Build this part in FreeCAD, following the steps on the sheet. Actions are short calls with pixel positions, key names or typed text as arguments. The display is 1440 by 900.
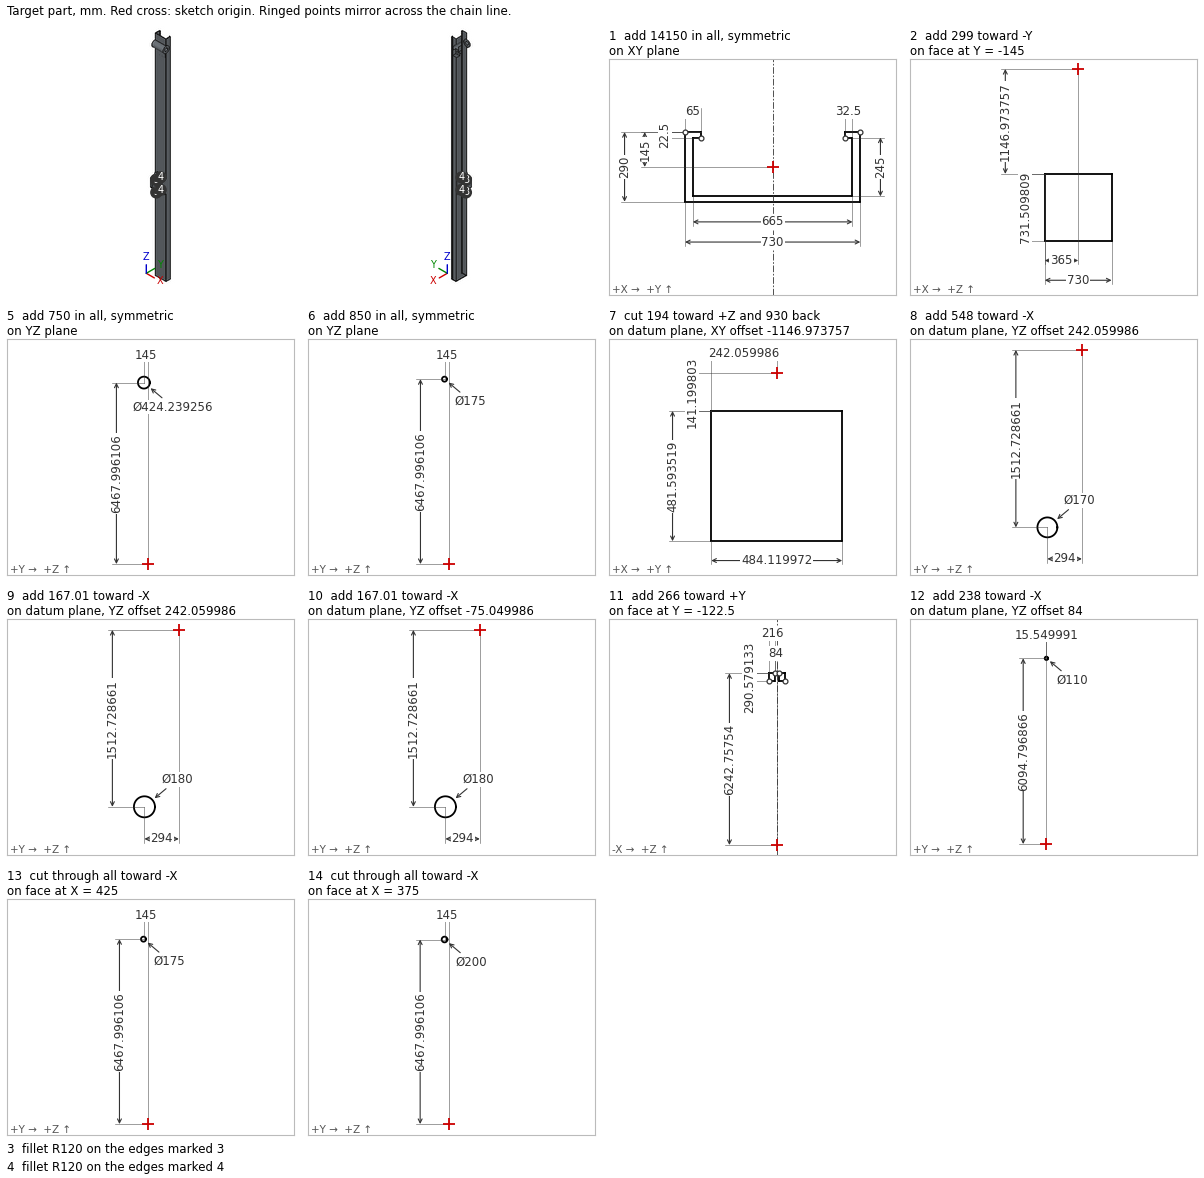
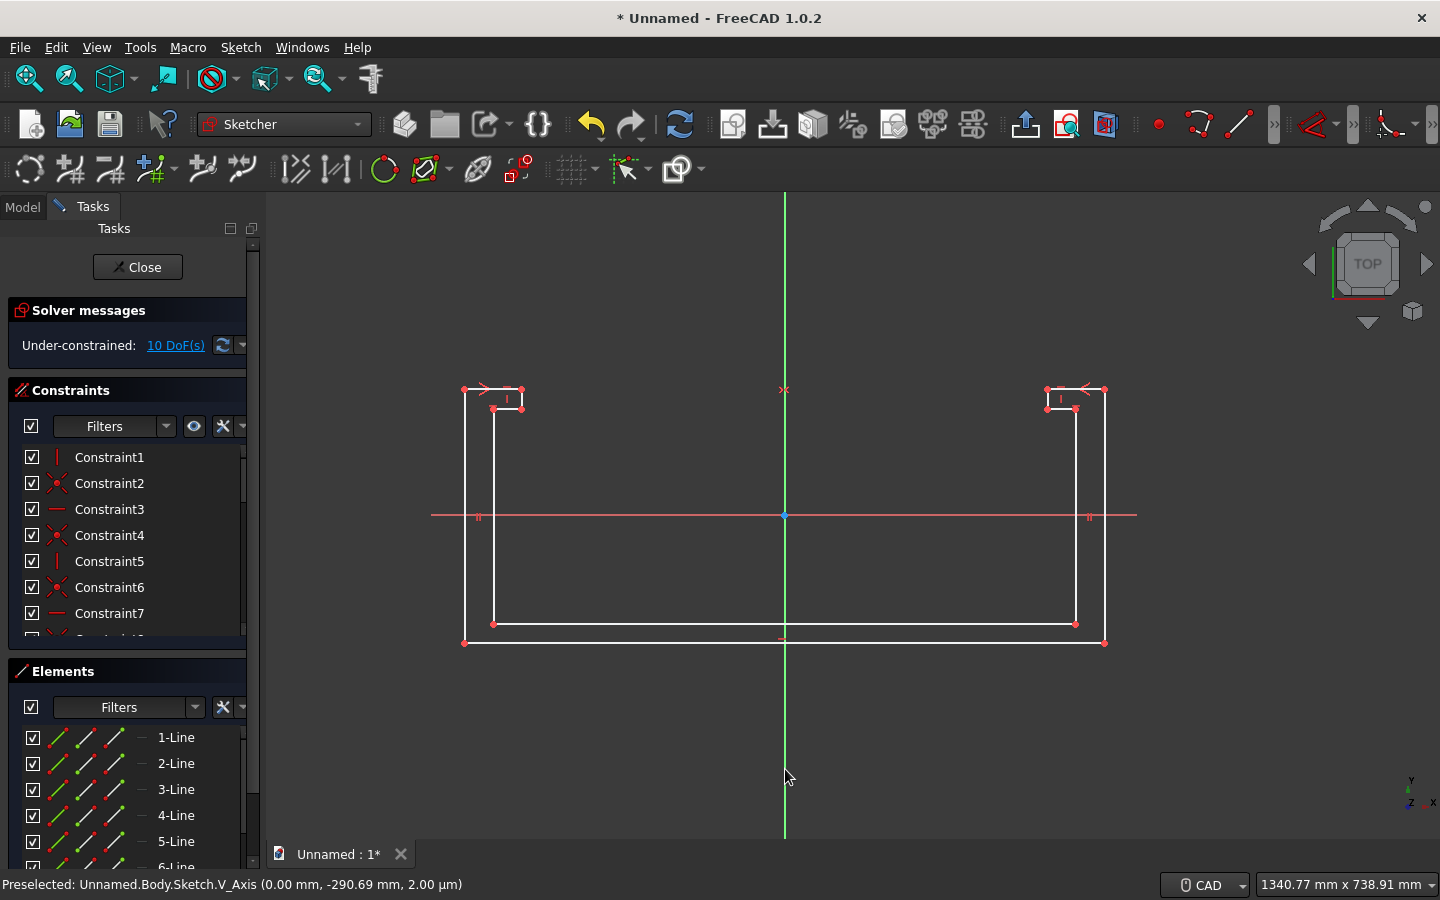
click(522, 409)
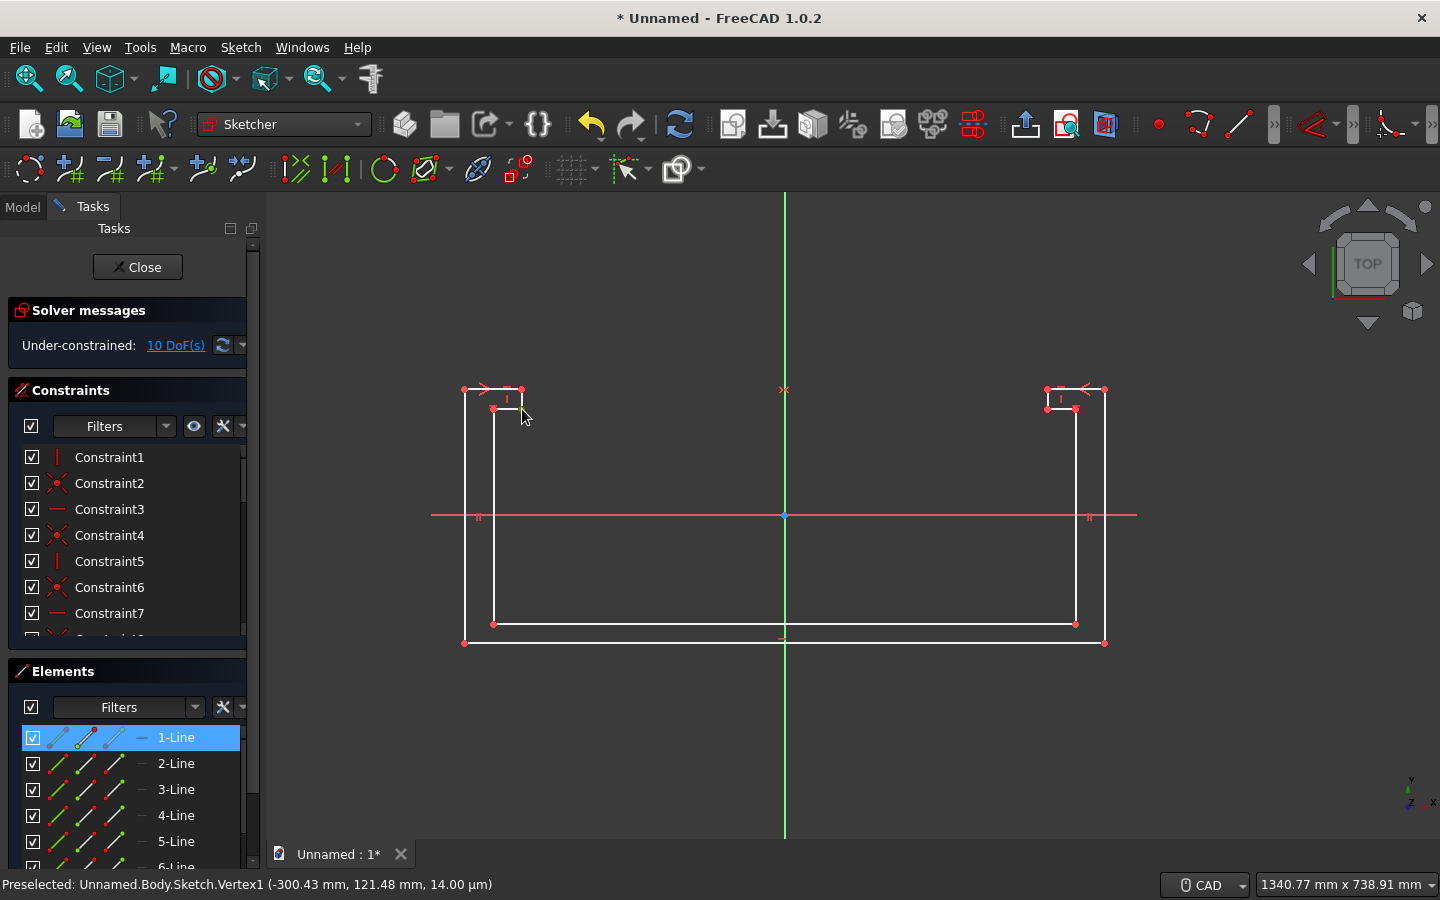
click(1048, 409)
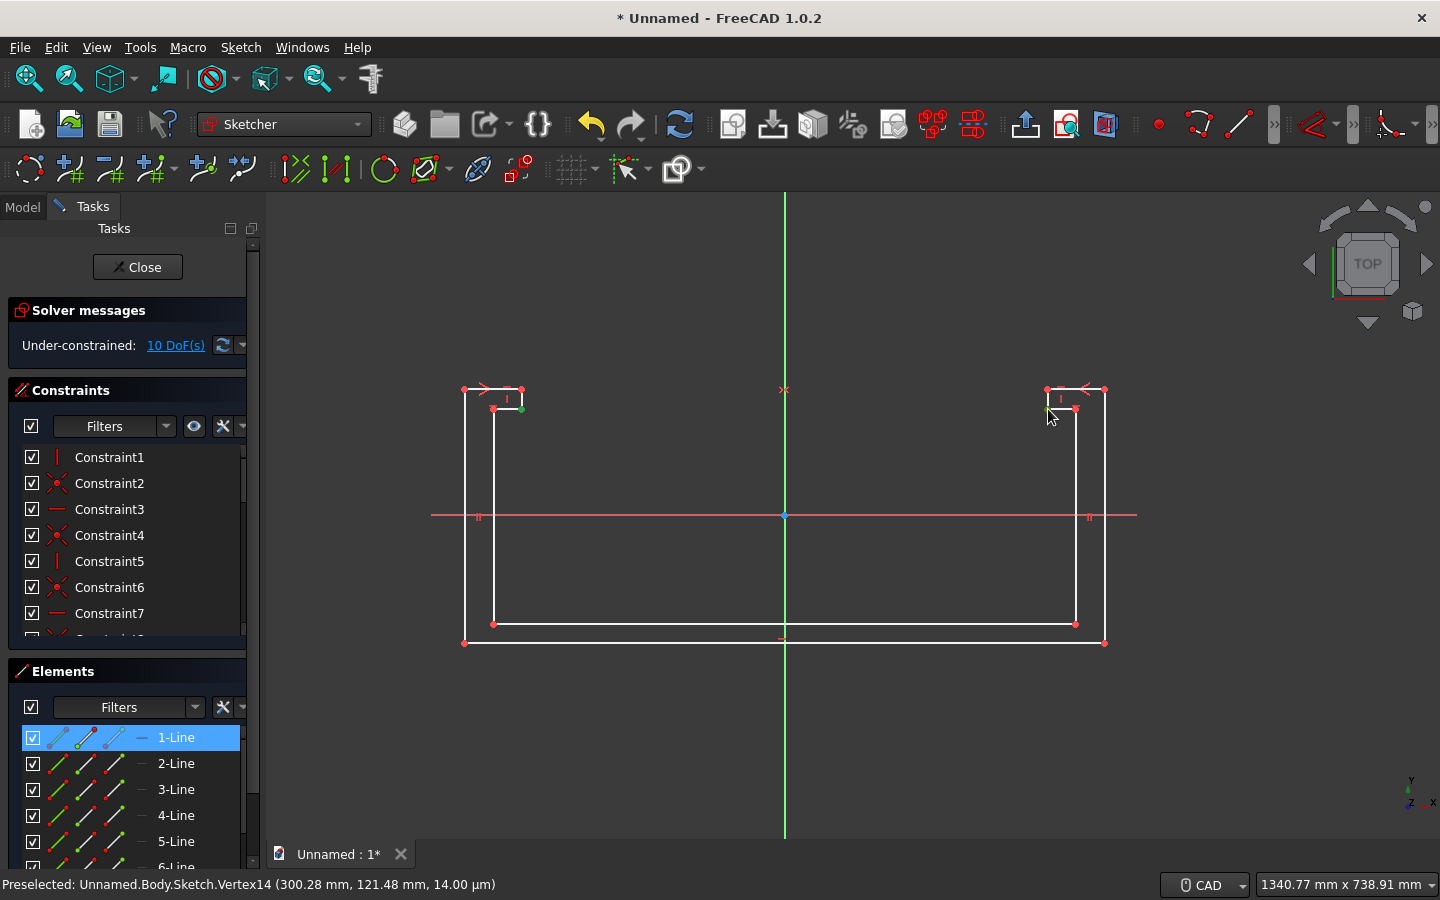
click(785, 769)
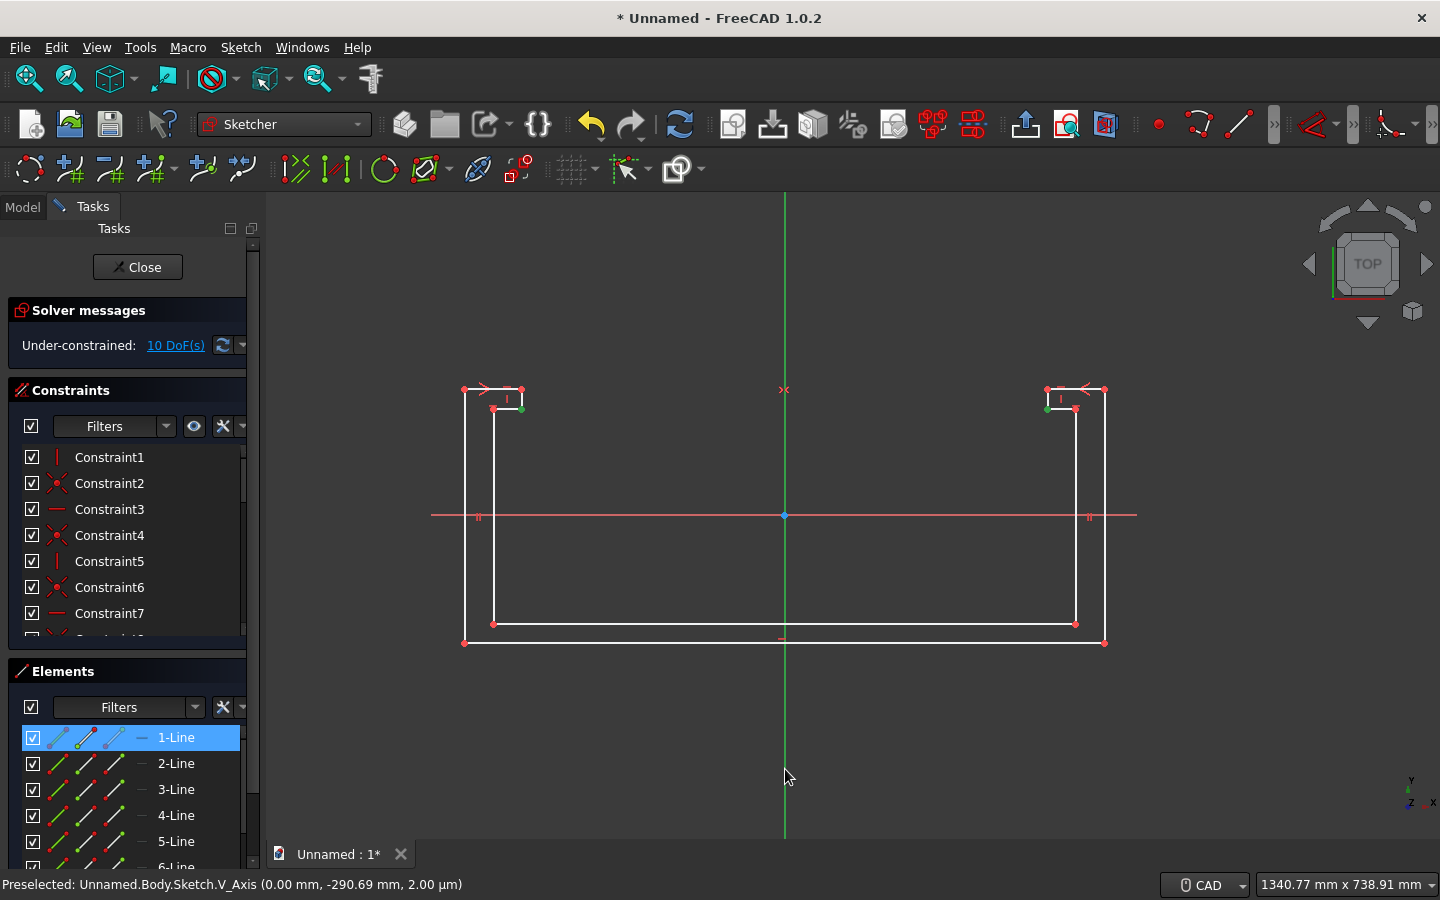
key(s)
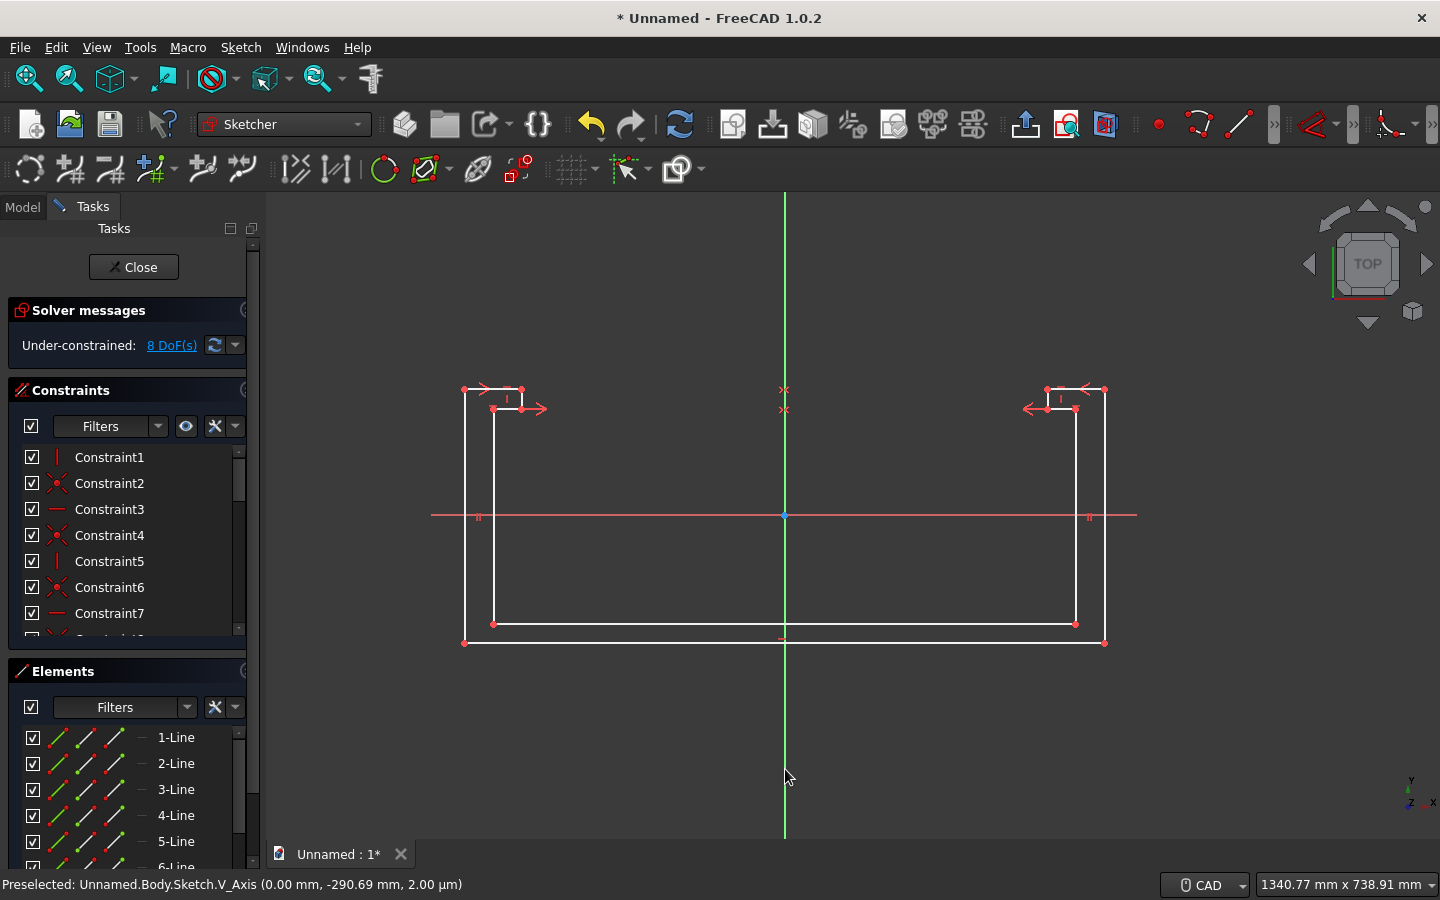
click(482, 389)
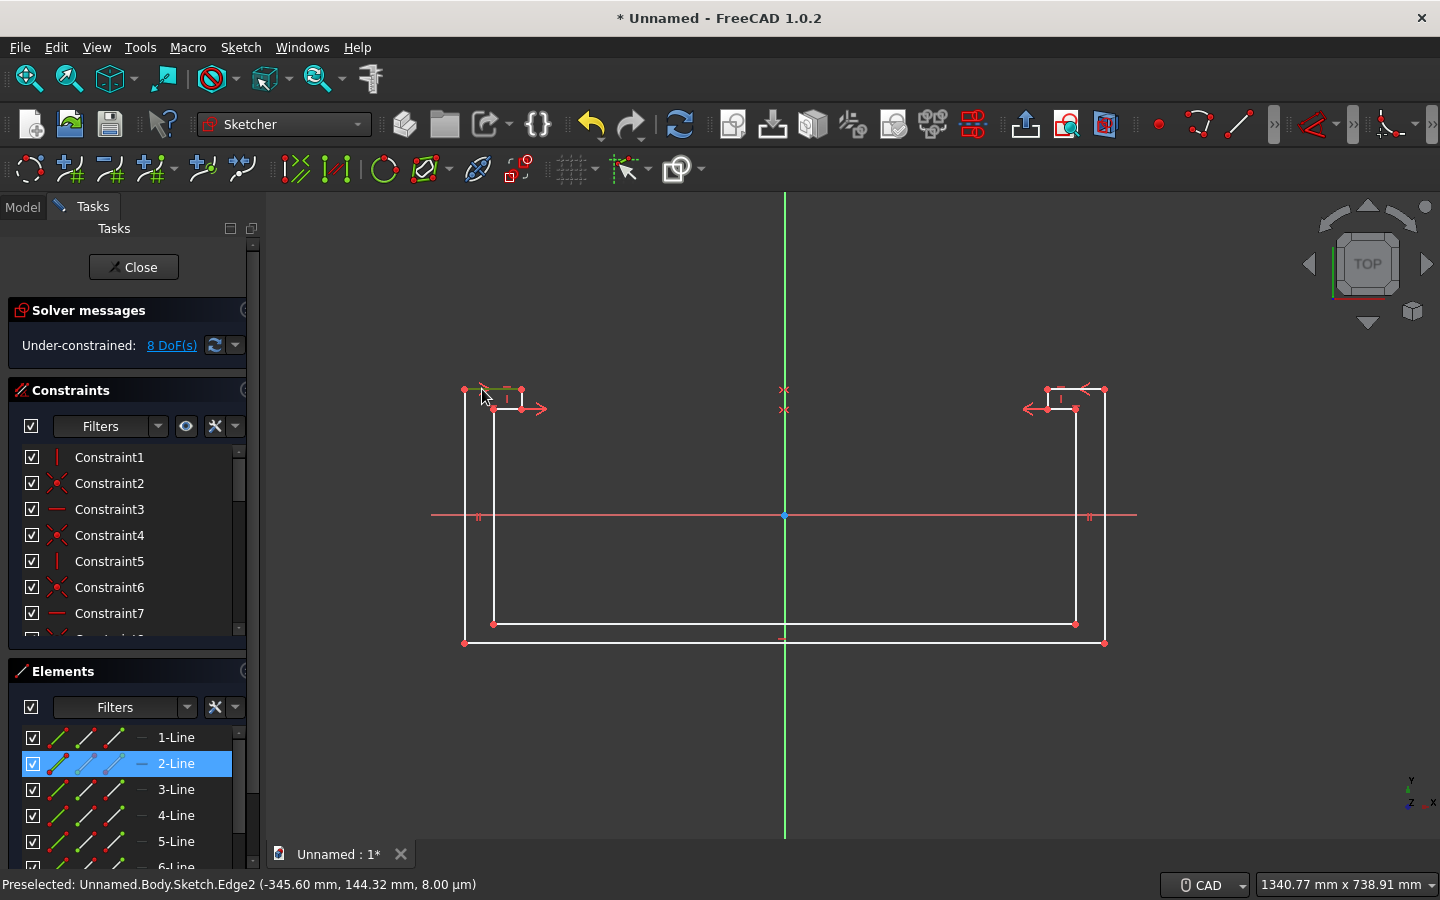
key(l)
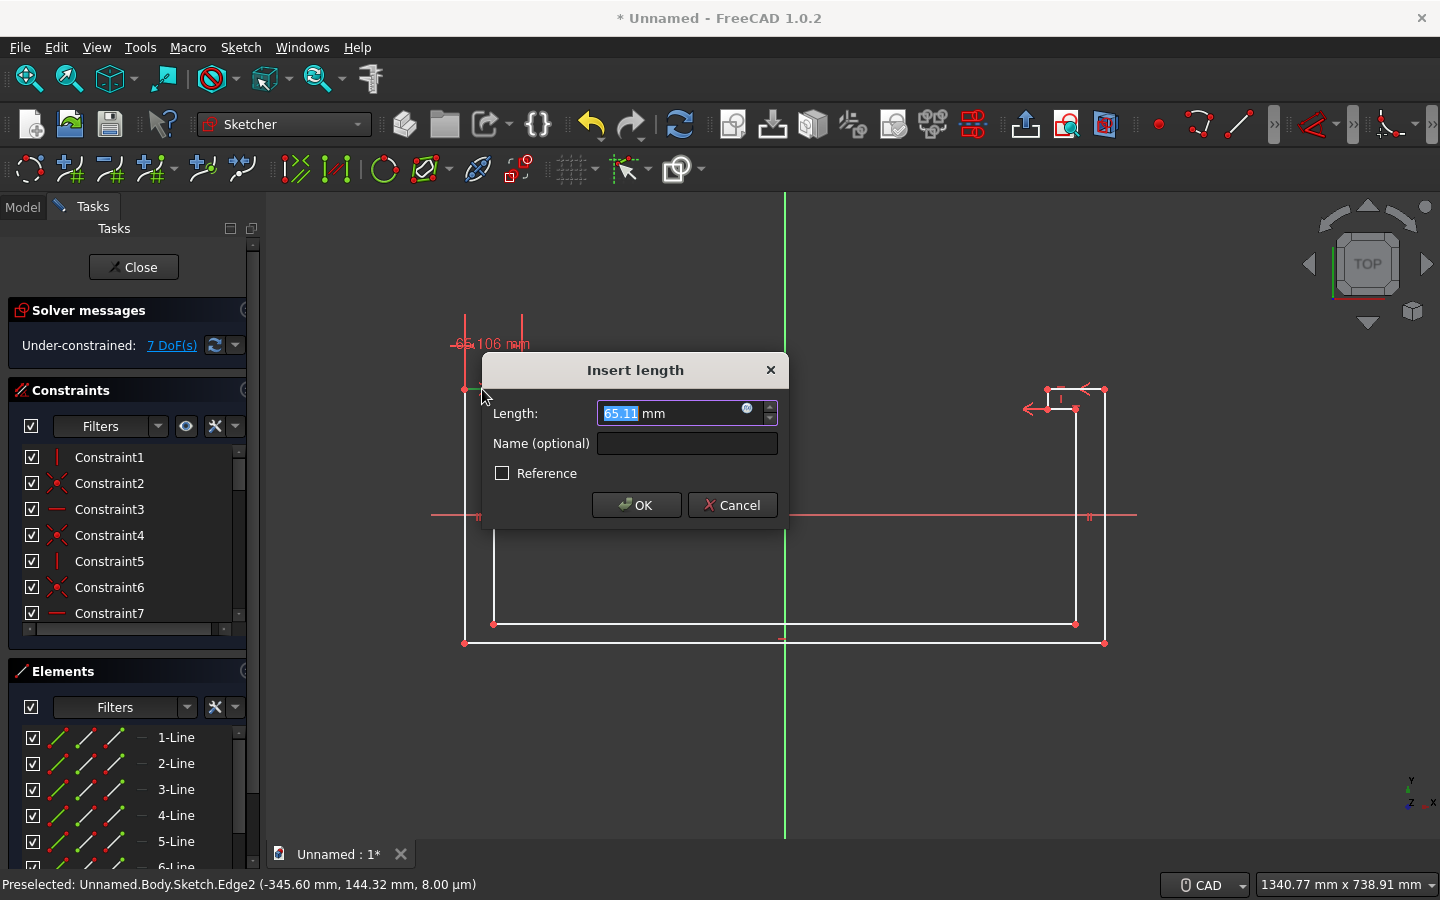
text(65)
key(Return)